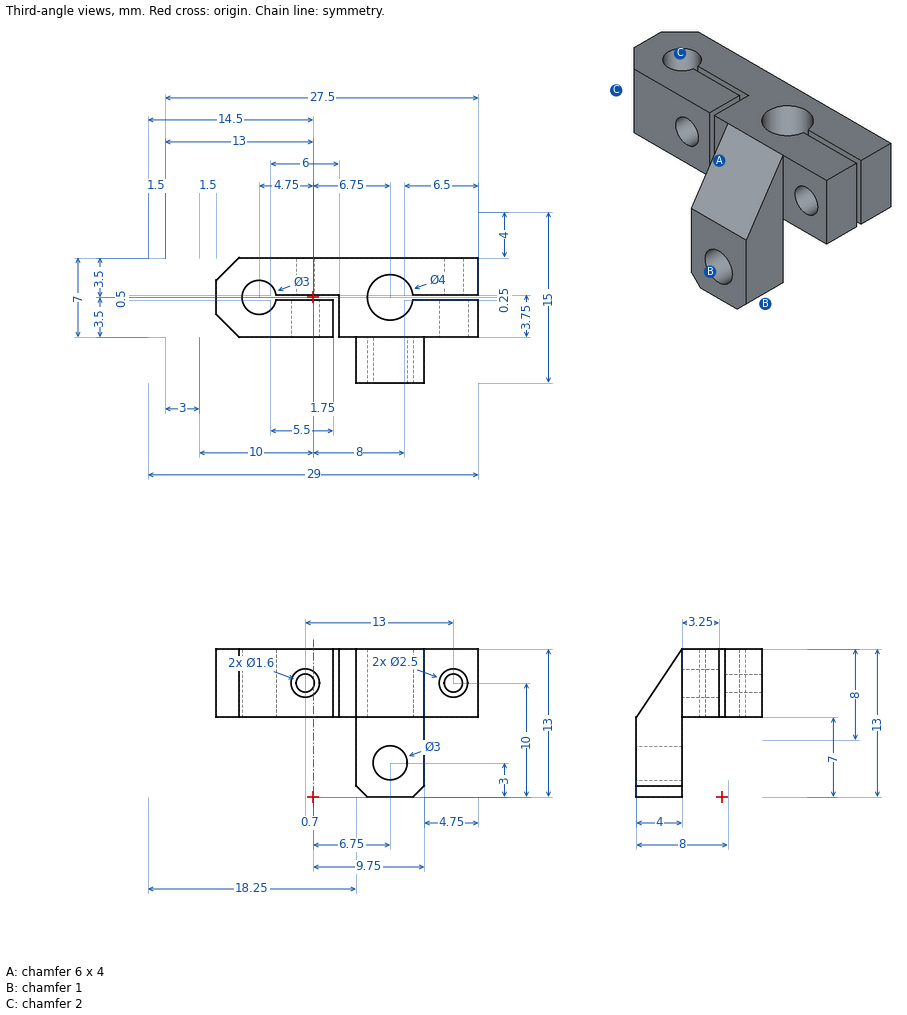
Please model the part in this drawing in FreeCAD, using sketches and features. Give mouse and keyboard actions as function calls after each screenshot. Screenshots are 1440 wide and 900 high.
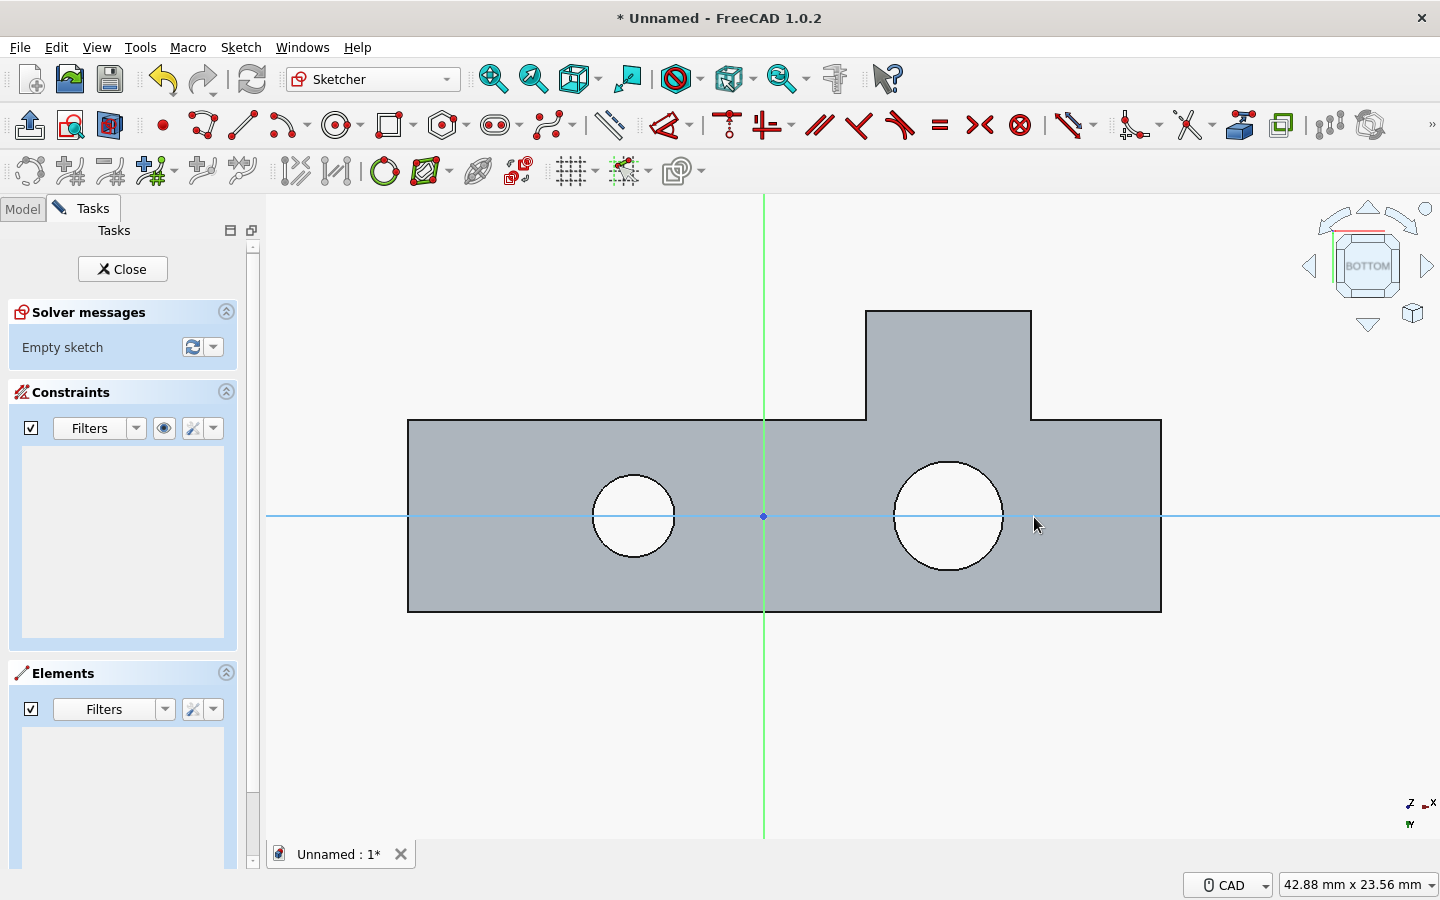
click(390, 126)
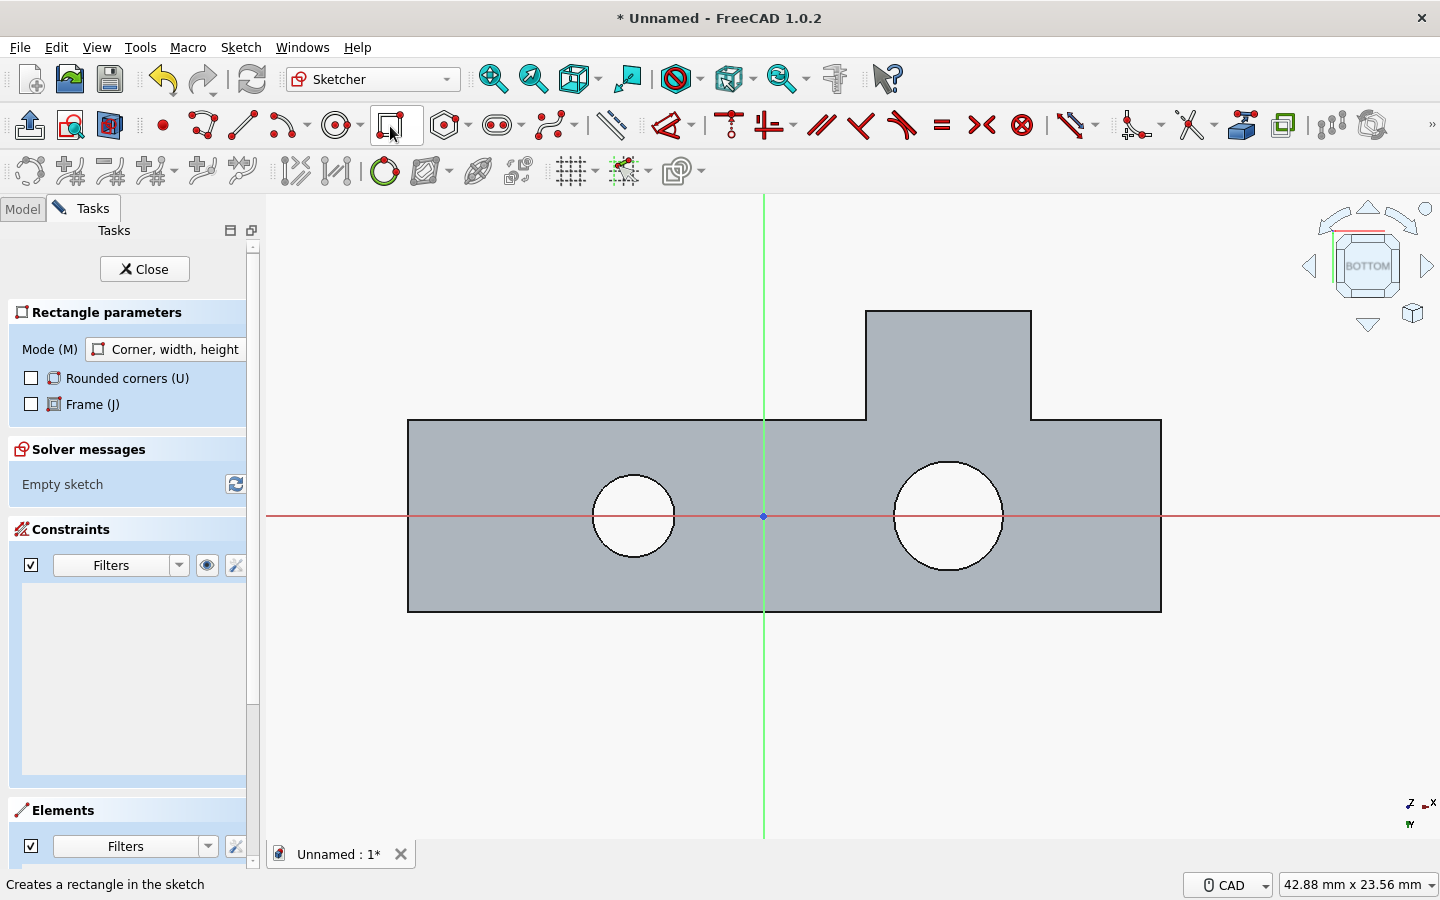
click(408, 420)
move(1161, 612)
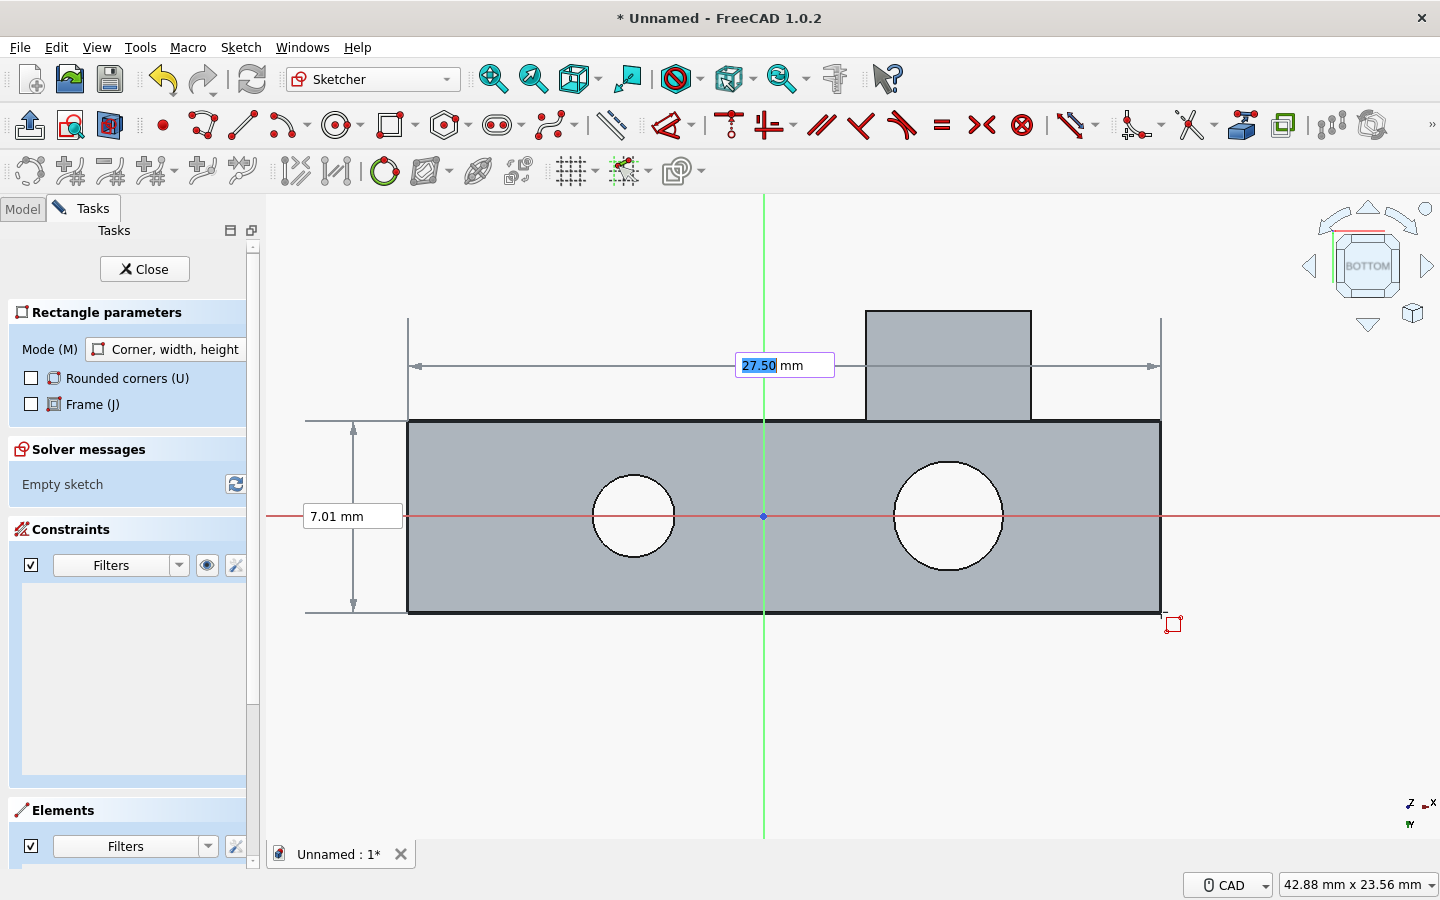
text(27.5)
key(Tab)
text(7)
key(Return)
key(Escape)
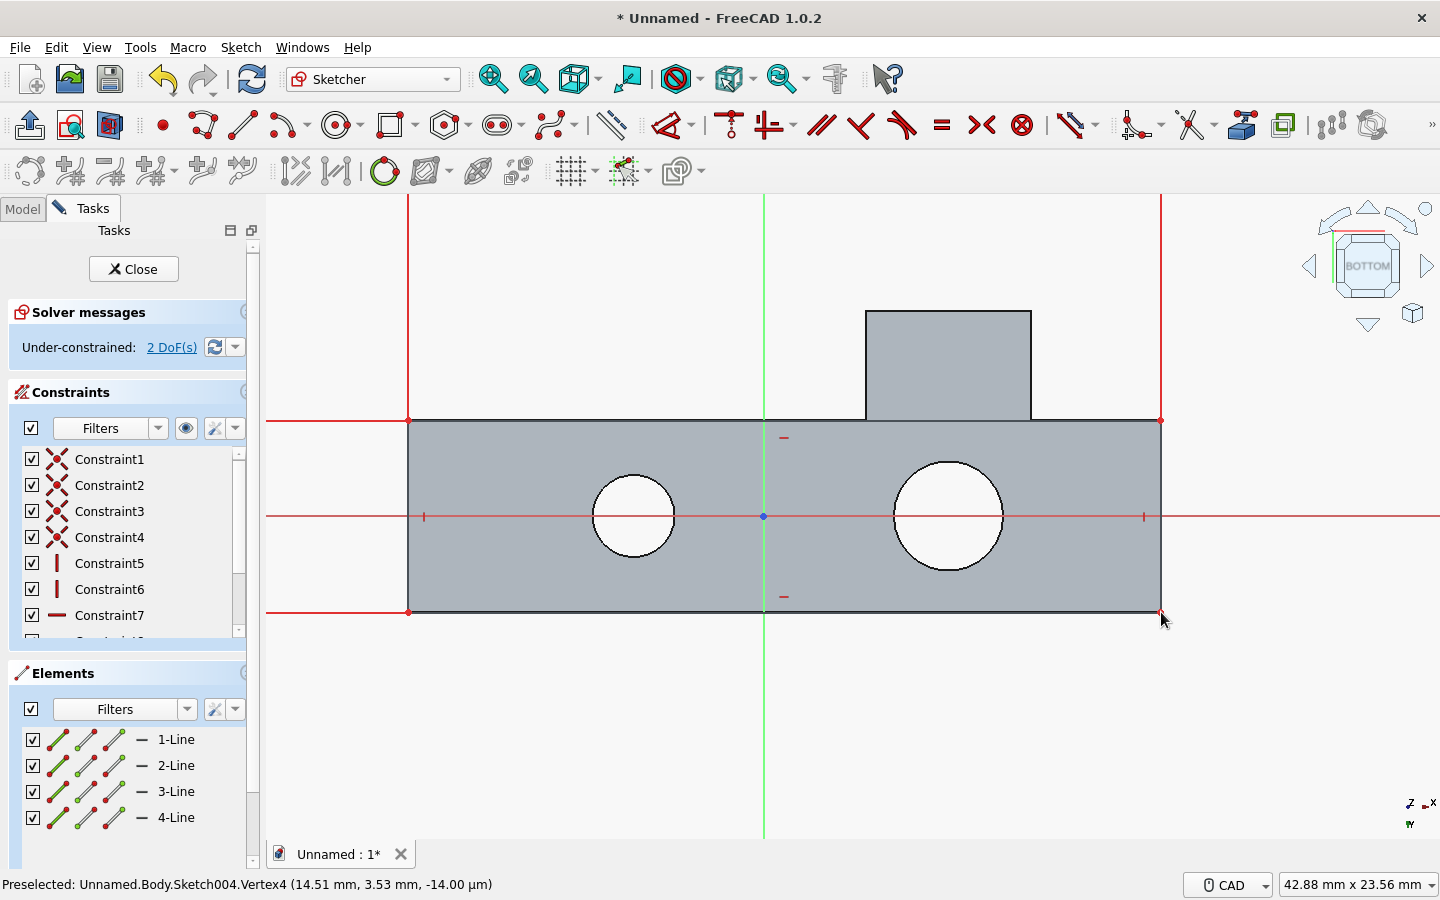
click(666, 126)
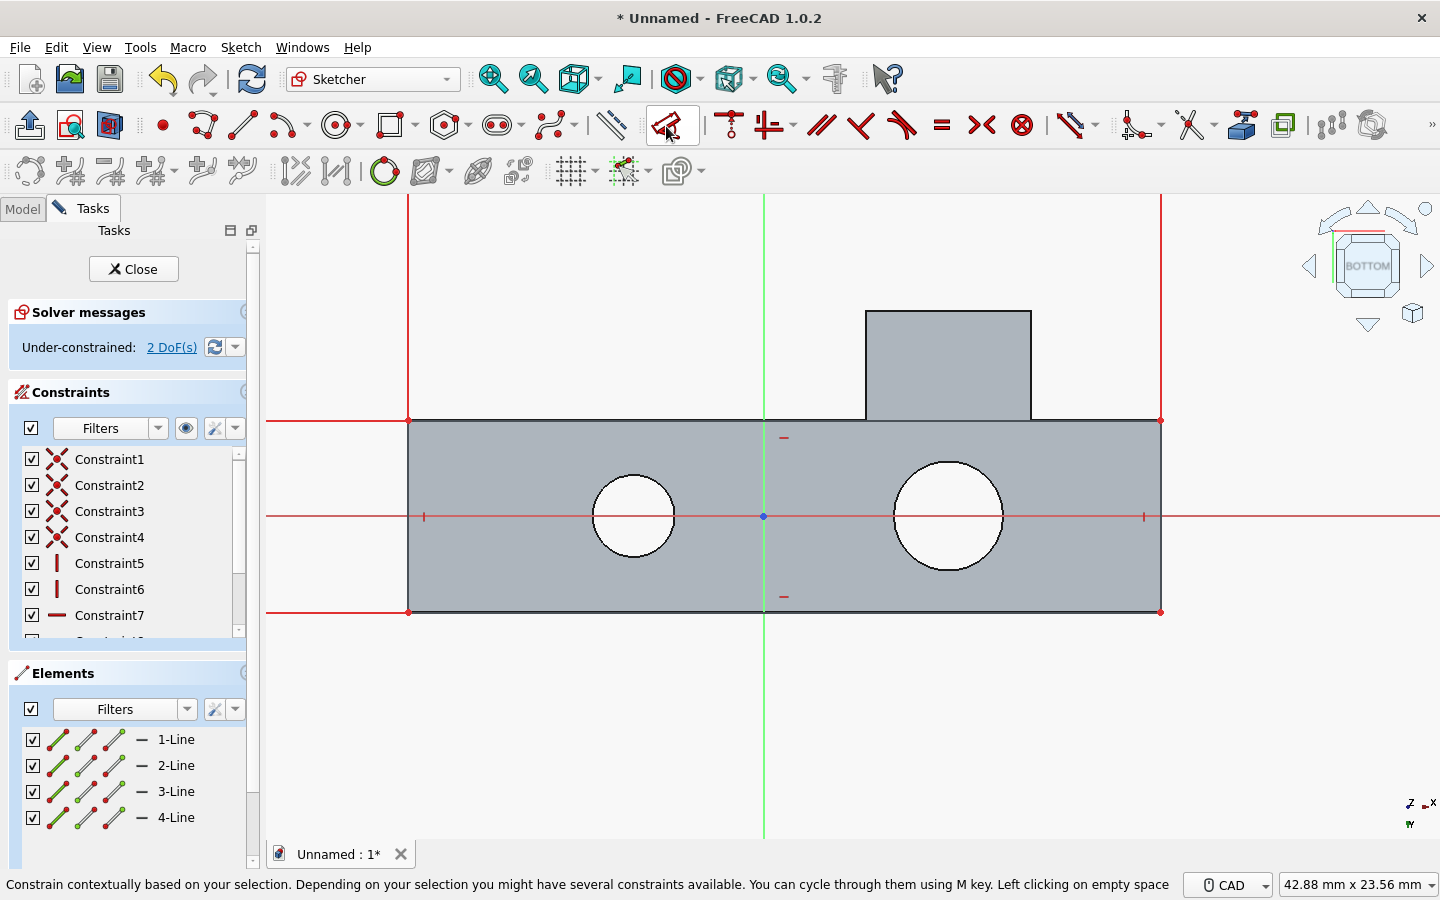
click(408, 421)
click(586, 387)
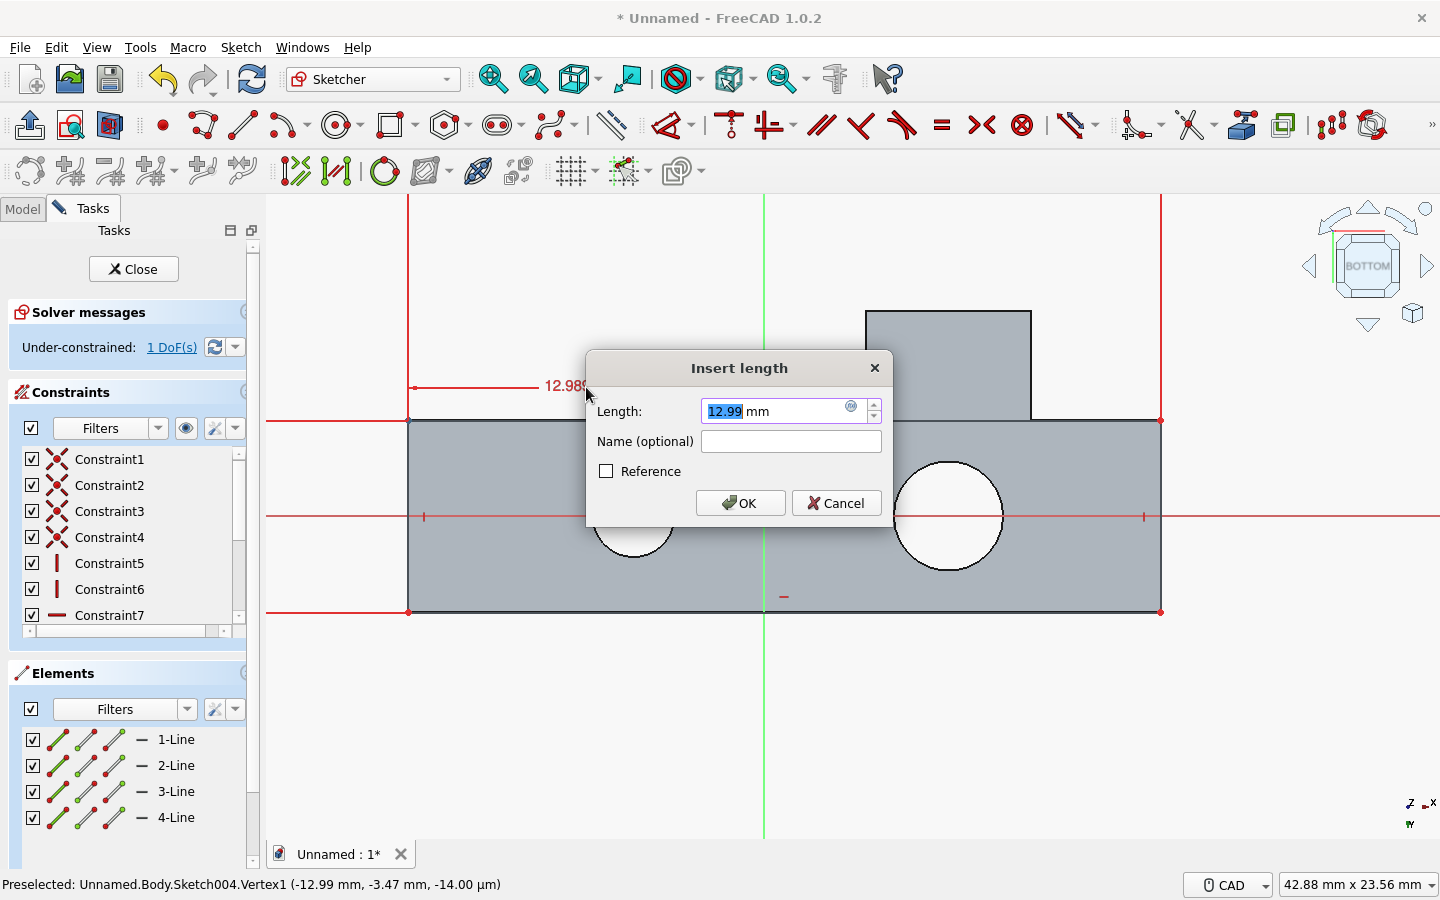
text(13)
key(Return)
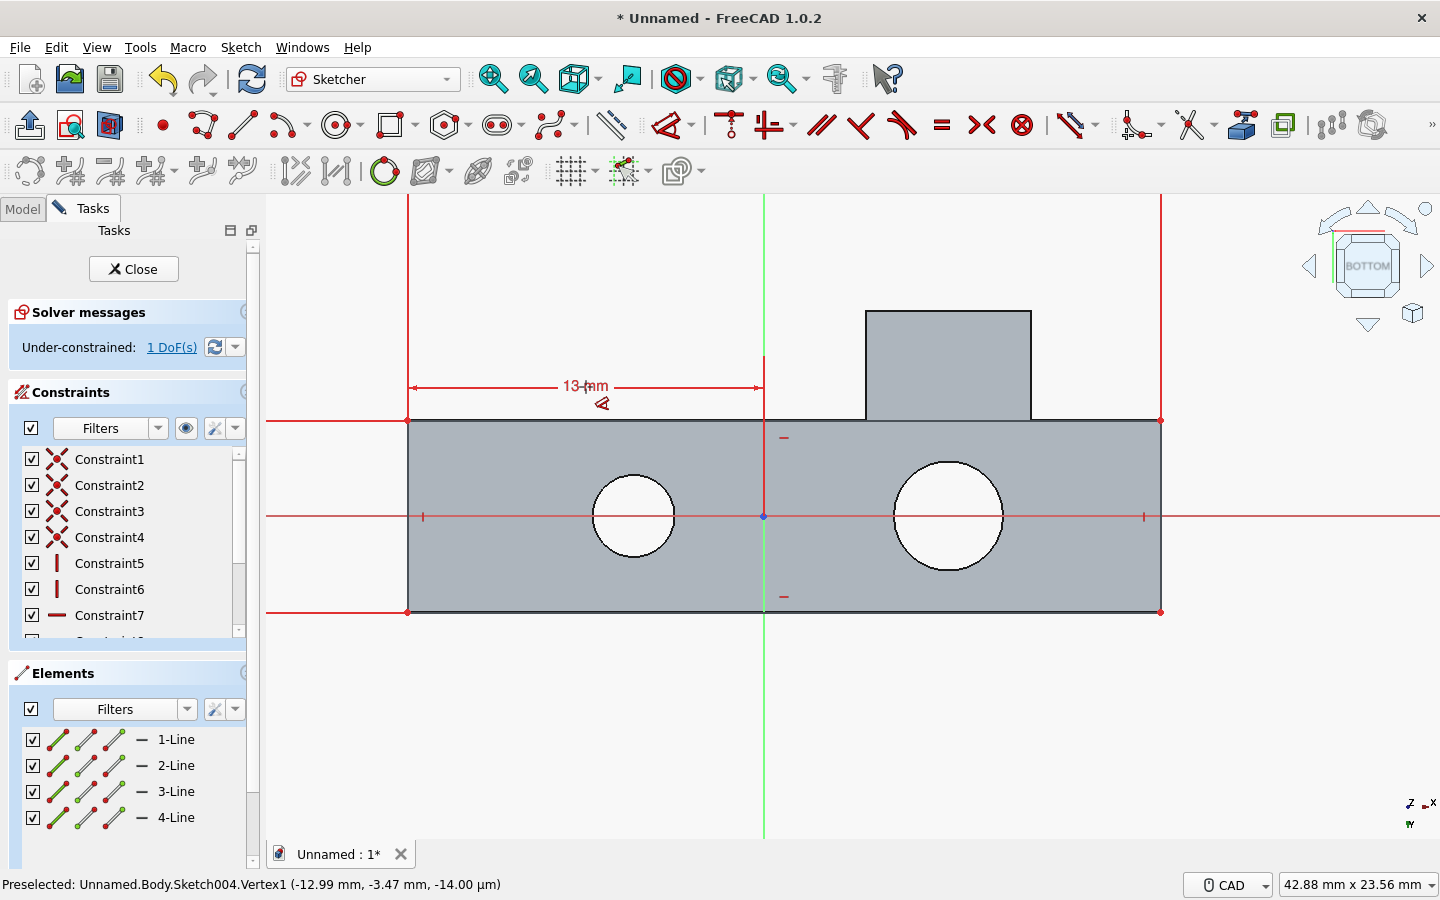
click(408, 421)
click(374, 469)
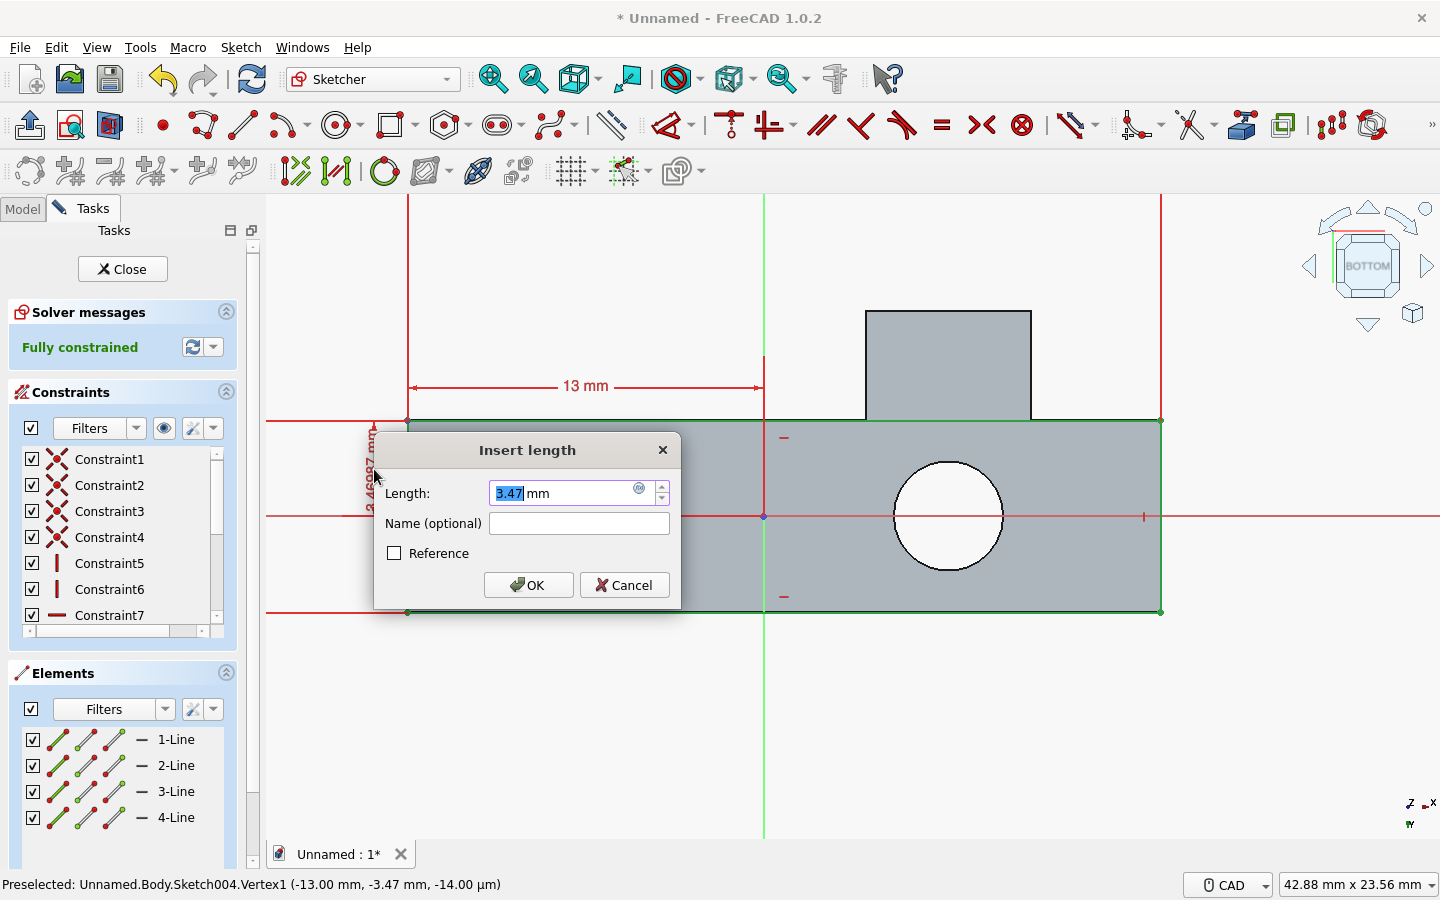
text(3.5)
key(Return)
key(Escape)